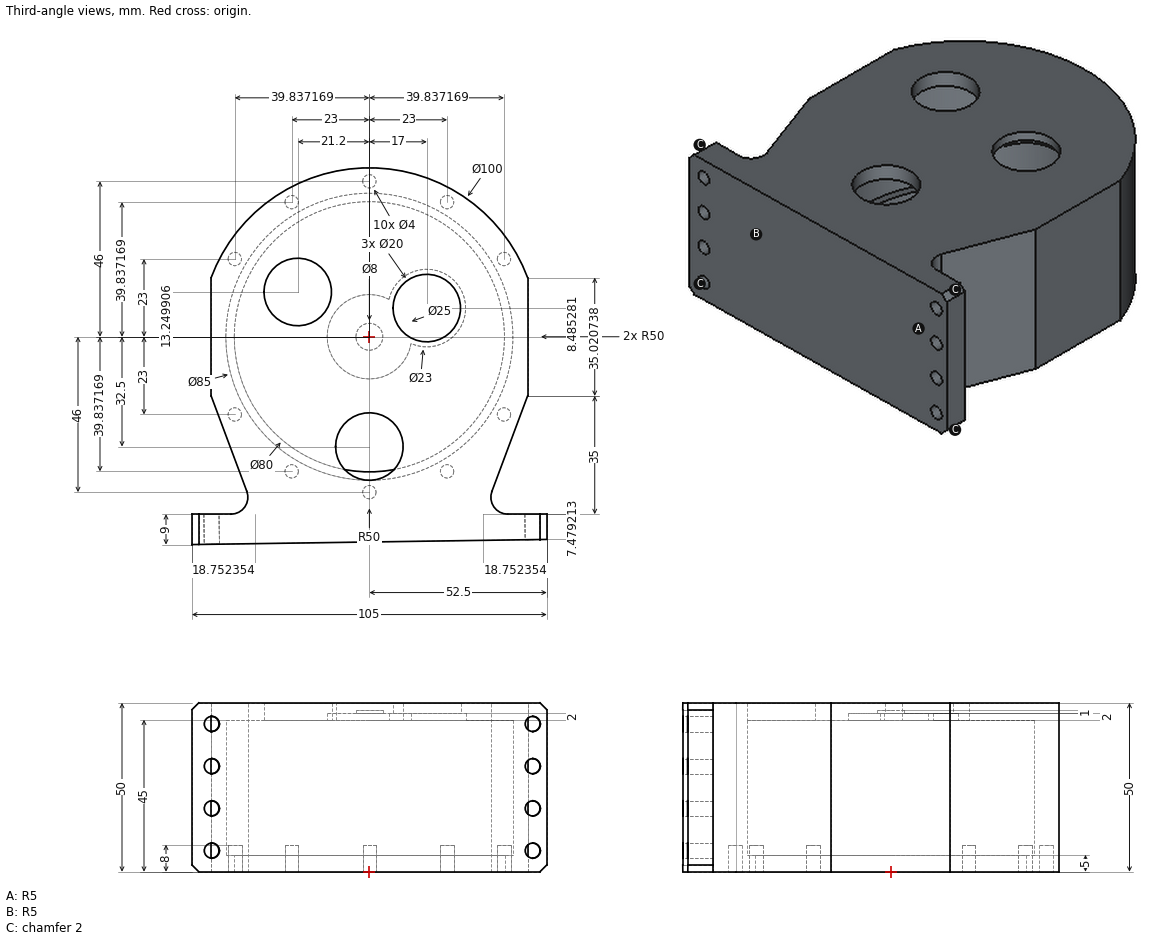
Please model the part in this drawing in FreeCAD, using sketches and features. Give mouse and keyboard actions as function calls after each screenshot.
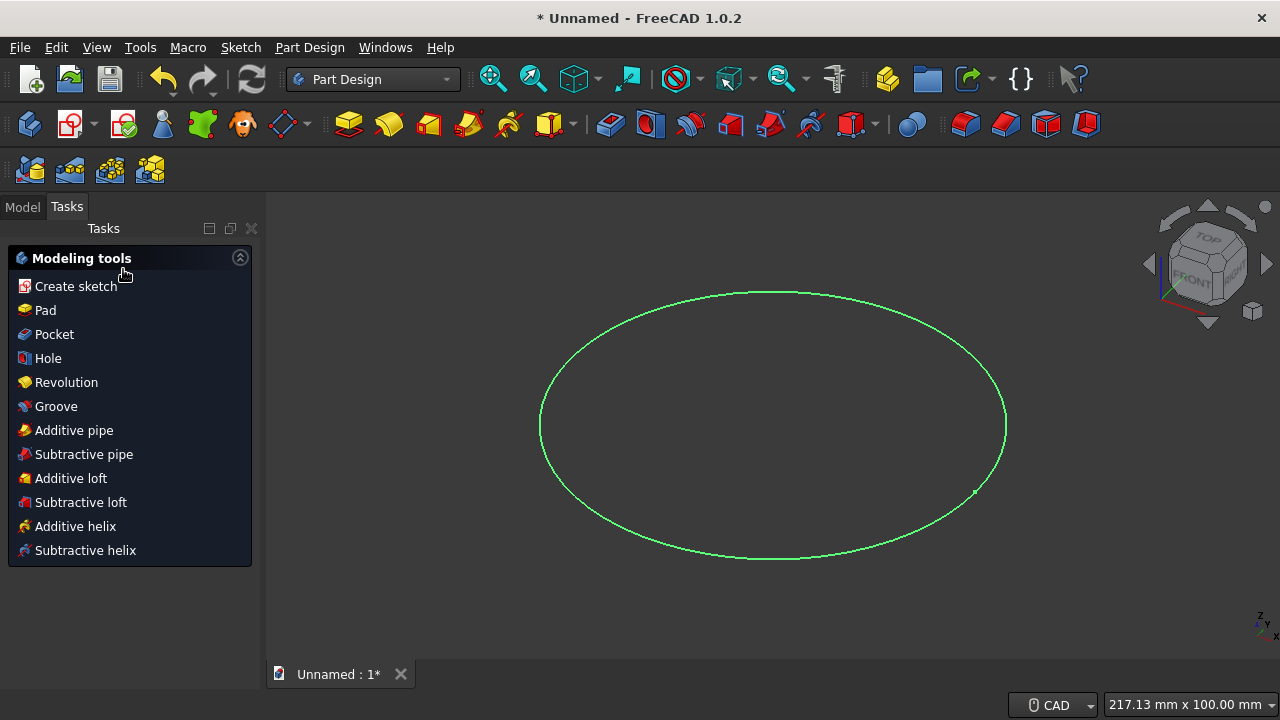
click(350, 124)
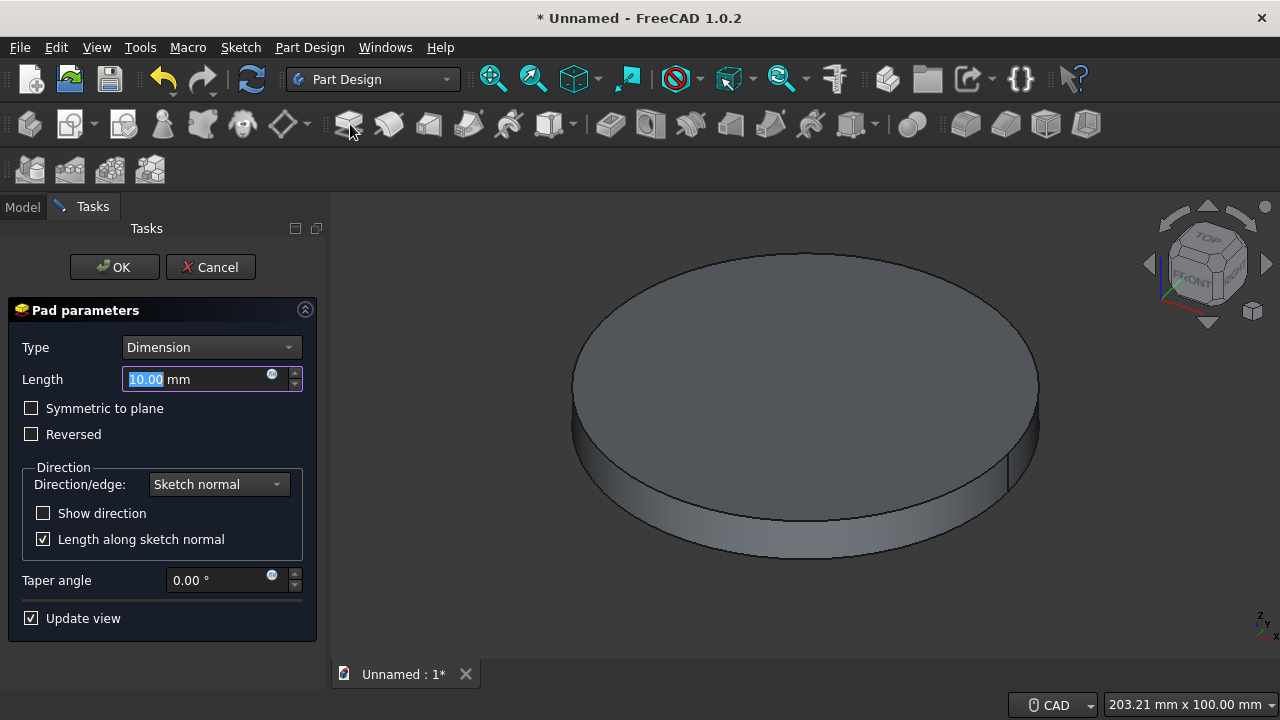
text(50)
key(Tab)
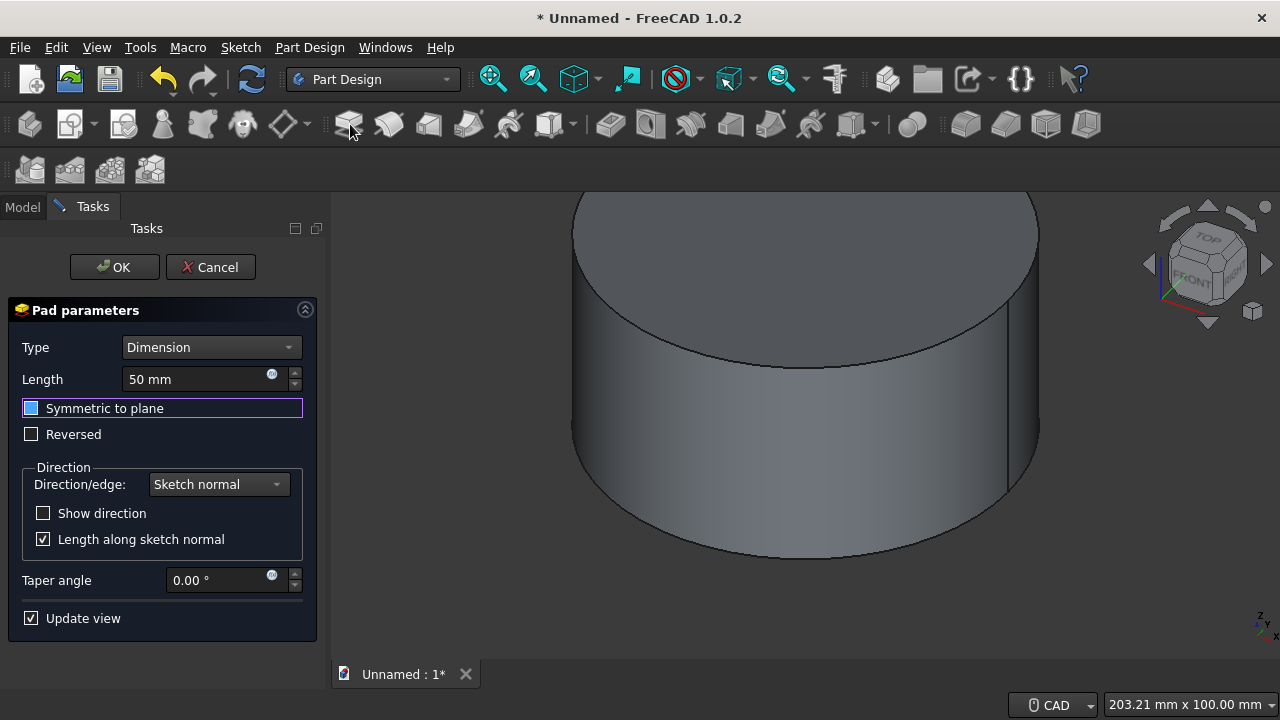
click(115, 267)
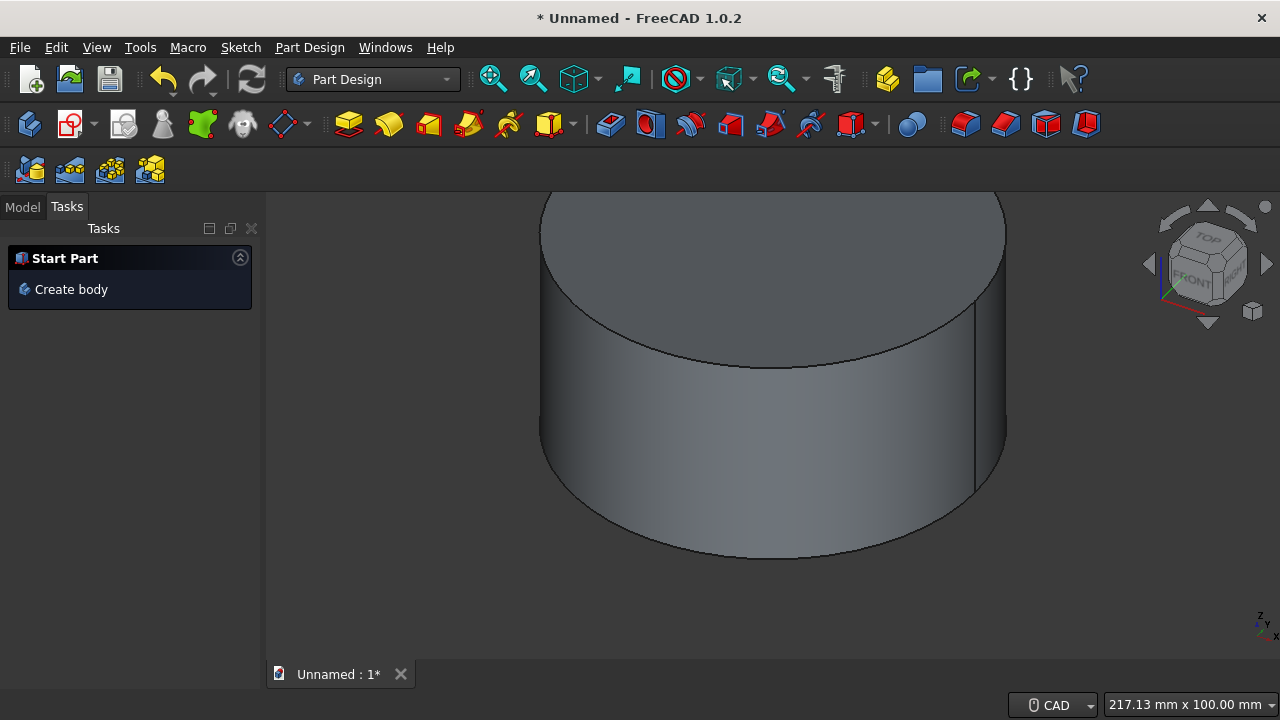
click(494, 80)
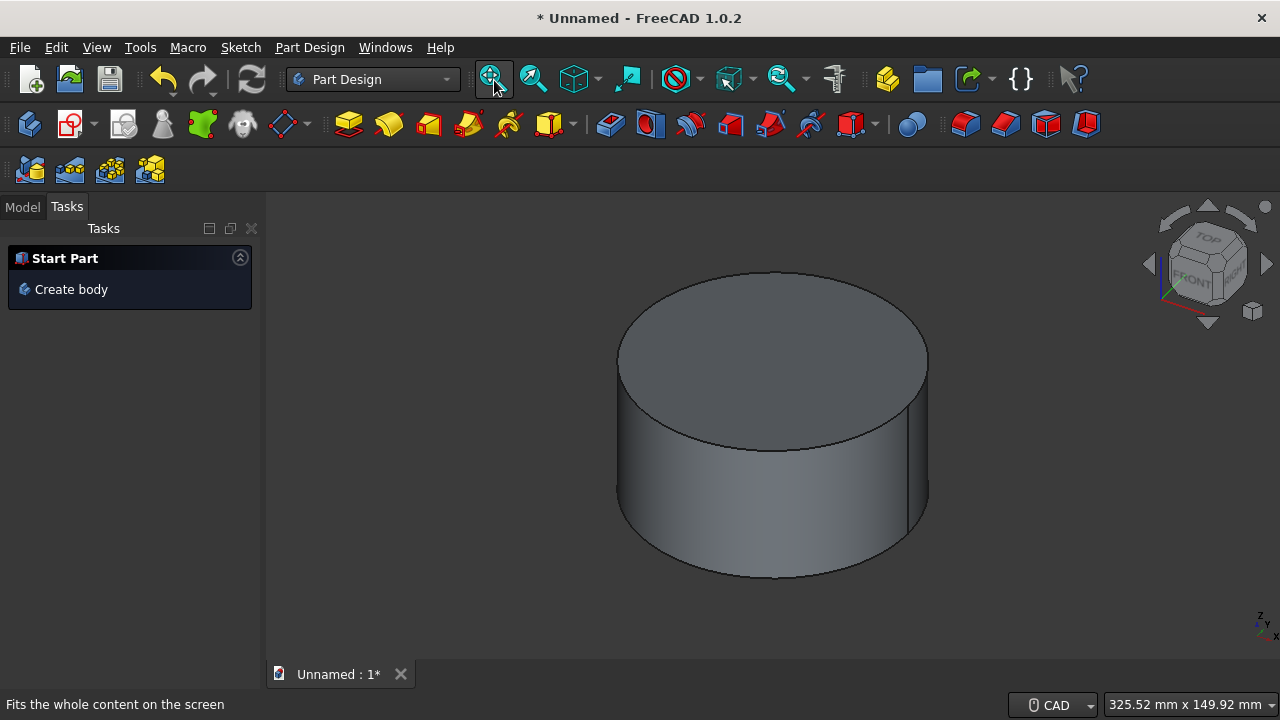
click(70, 124)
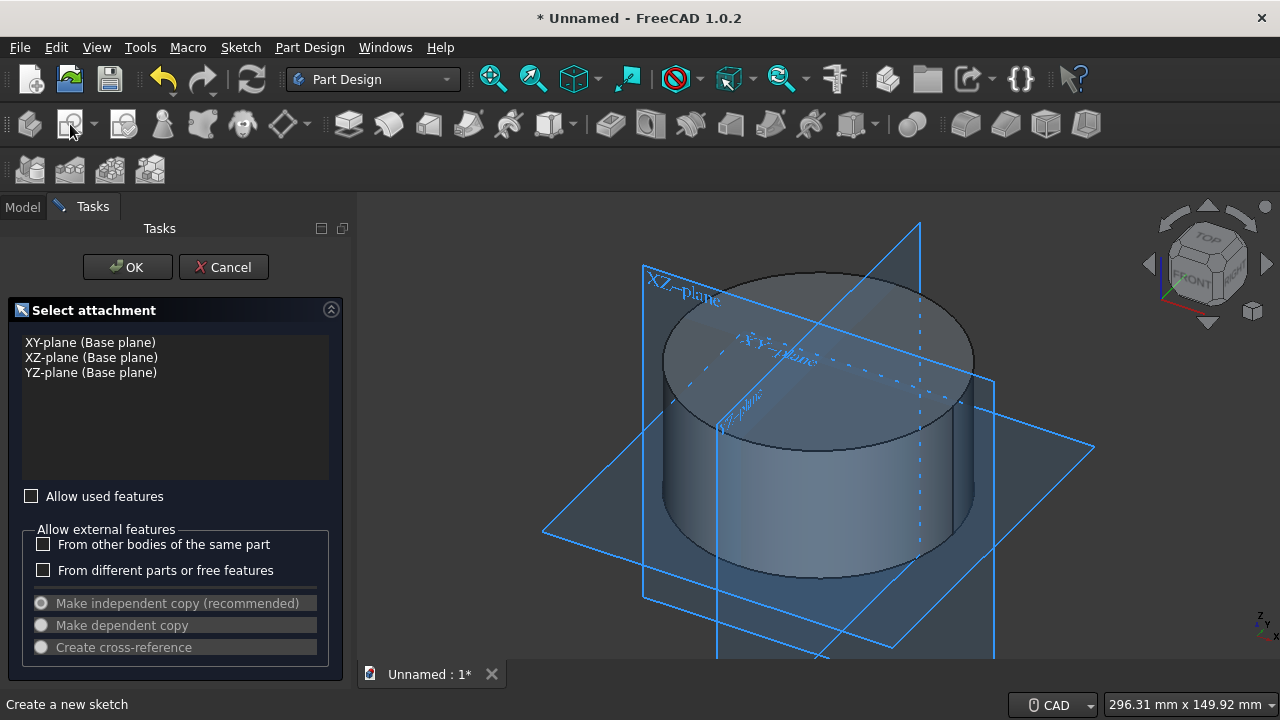
click(82, 342)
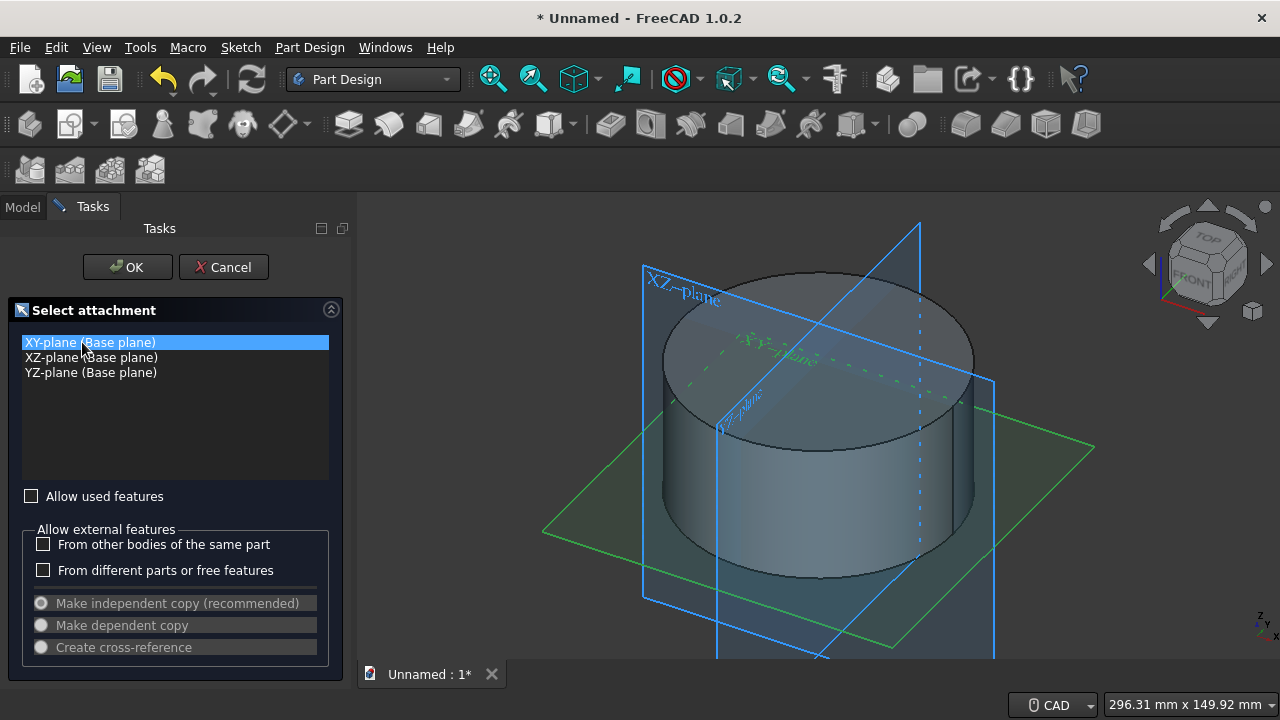
click(128, 267)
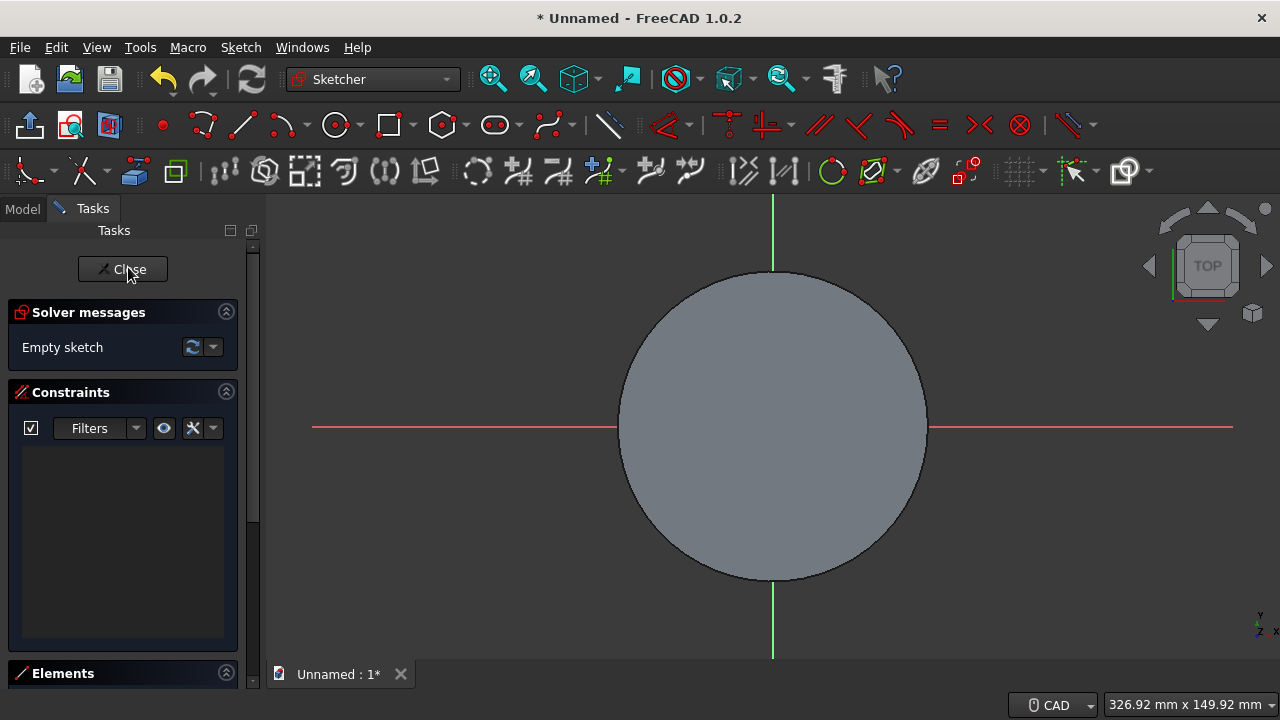
key(q)
key(s)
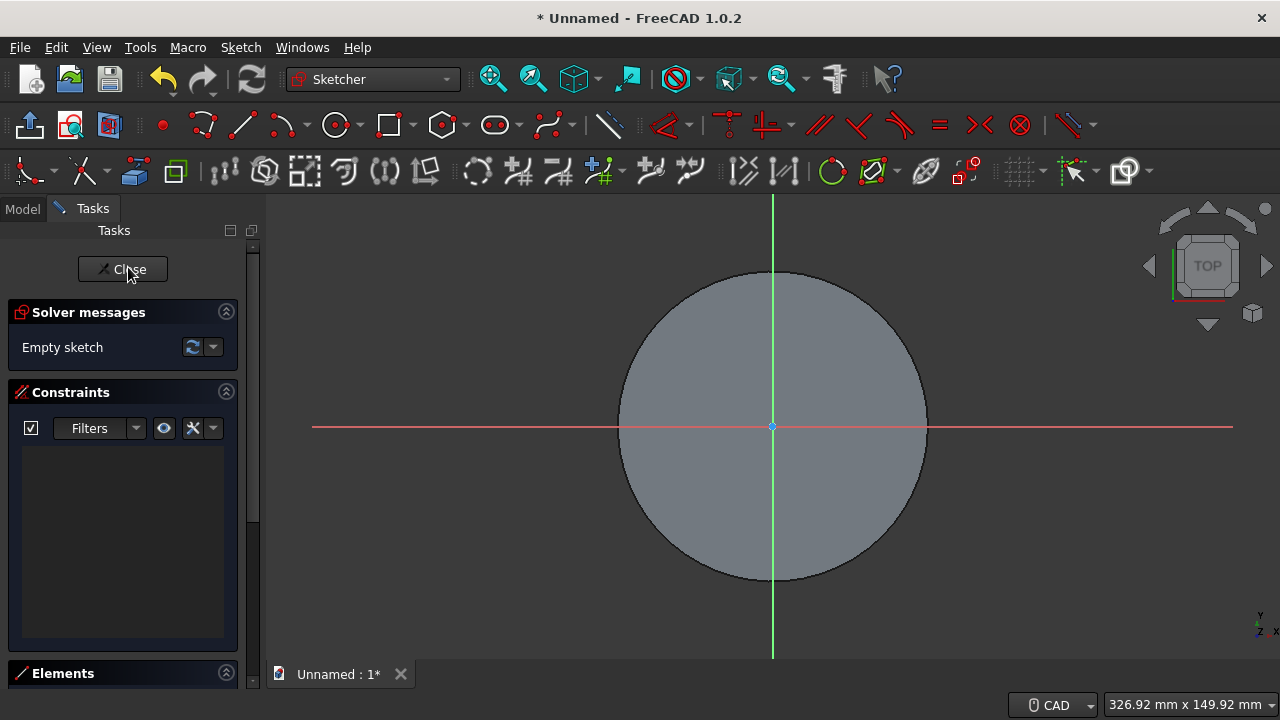
click(336, 126)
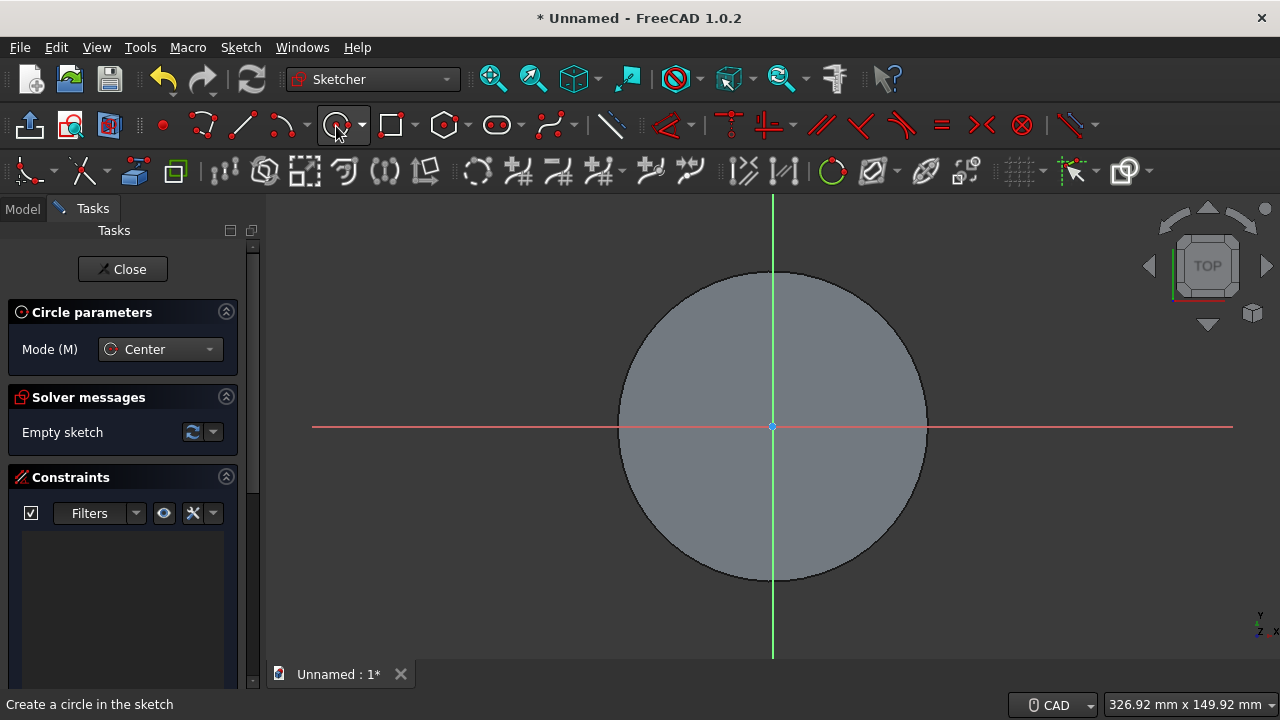
click(773, 426)
click(866, 333)
key(Escape)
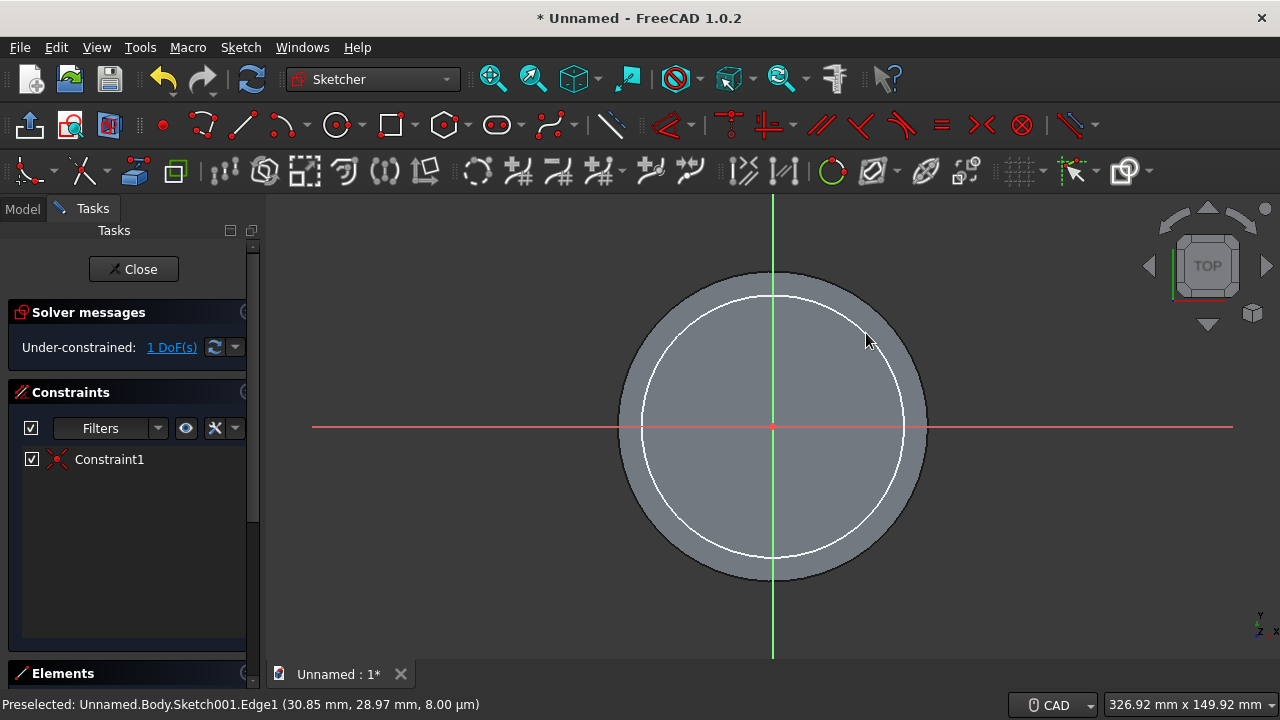
click(666, 126)